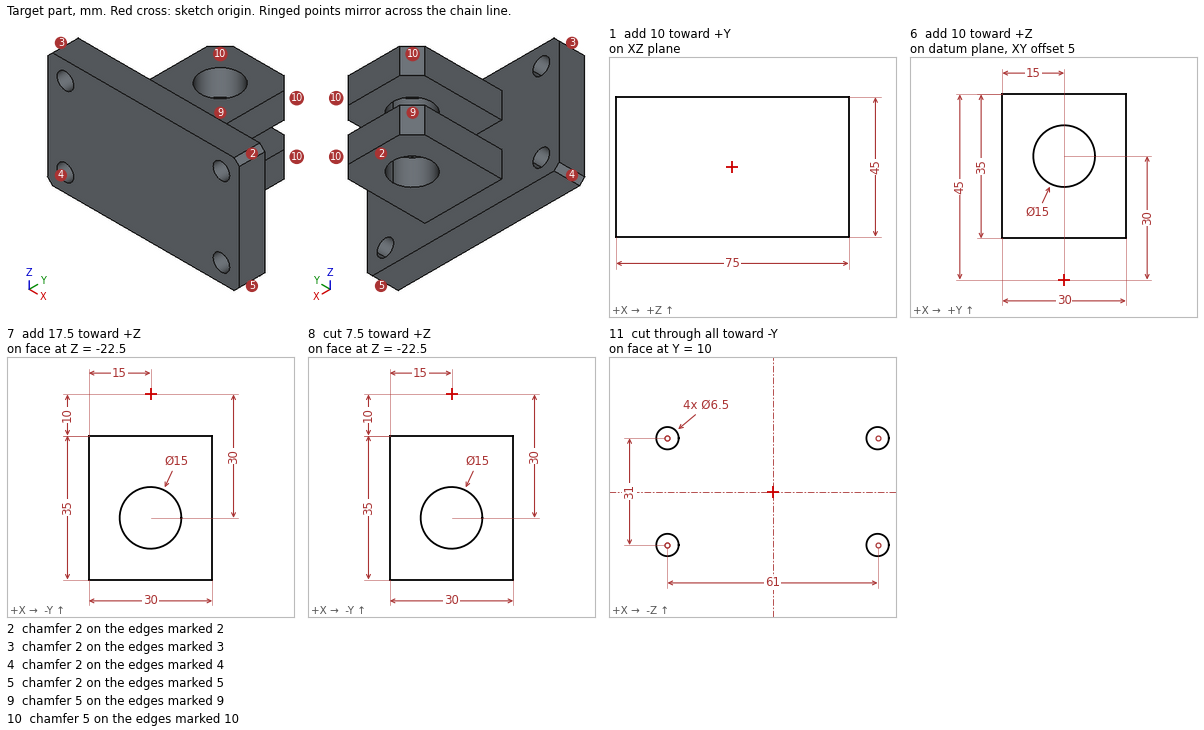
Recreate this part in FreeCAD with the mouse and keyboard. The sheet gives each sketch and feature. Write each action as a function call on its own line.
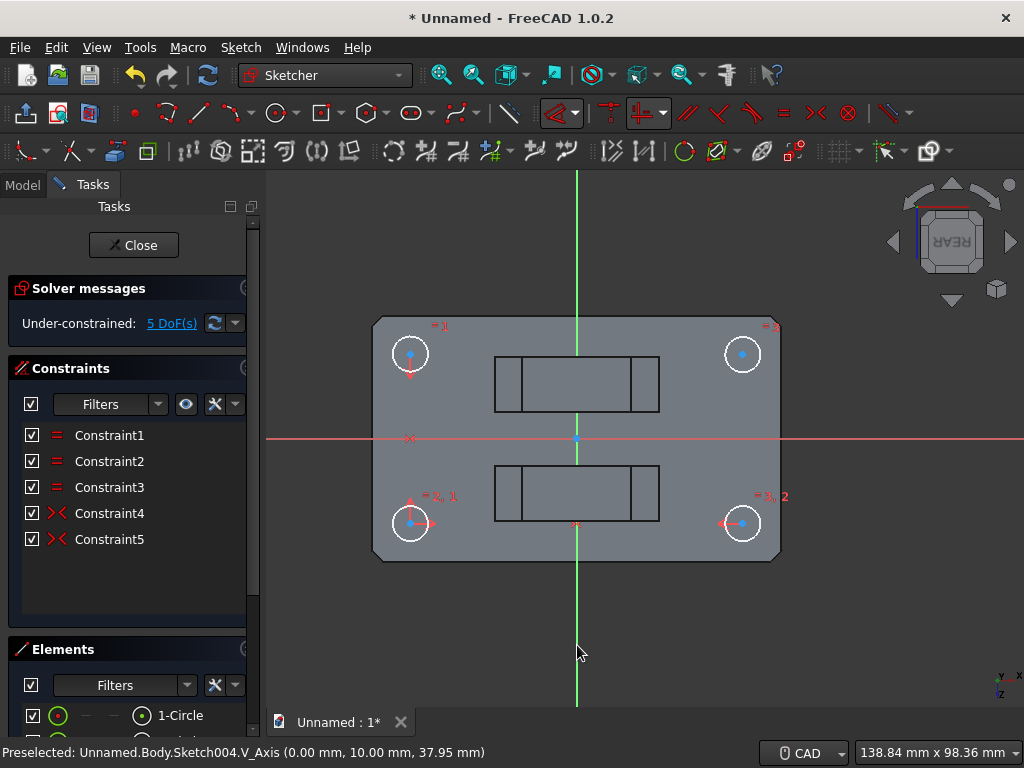
click(410, 354)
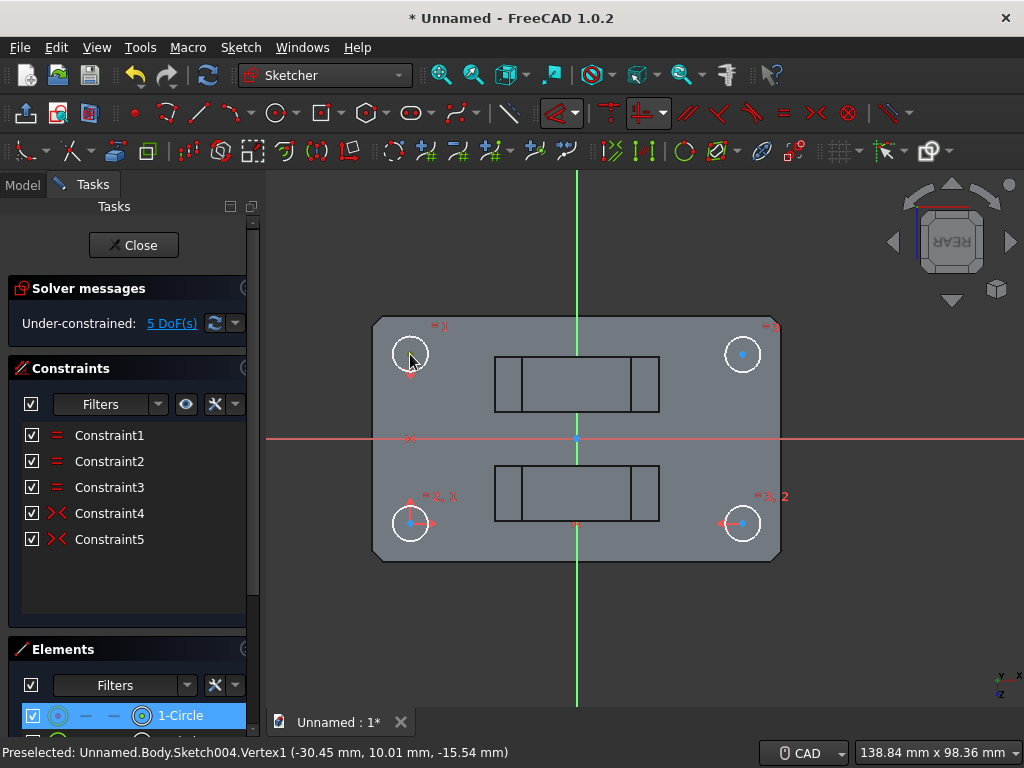
click(743, 355)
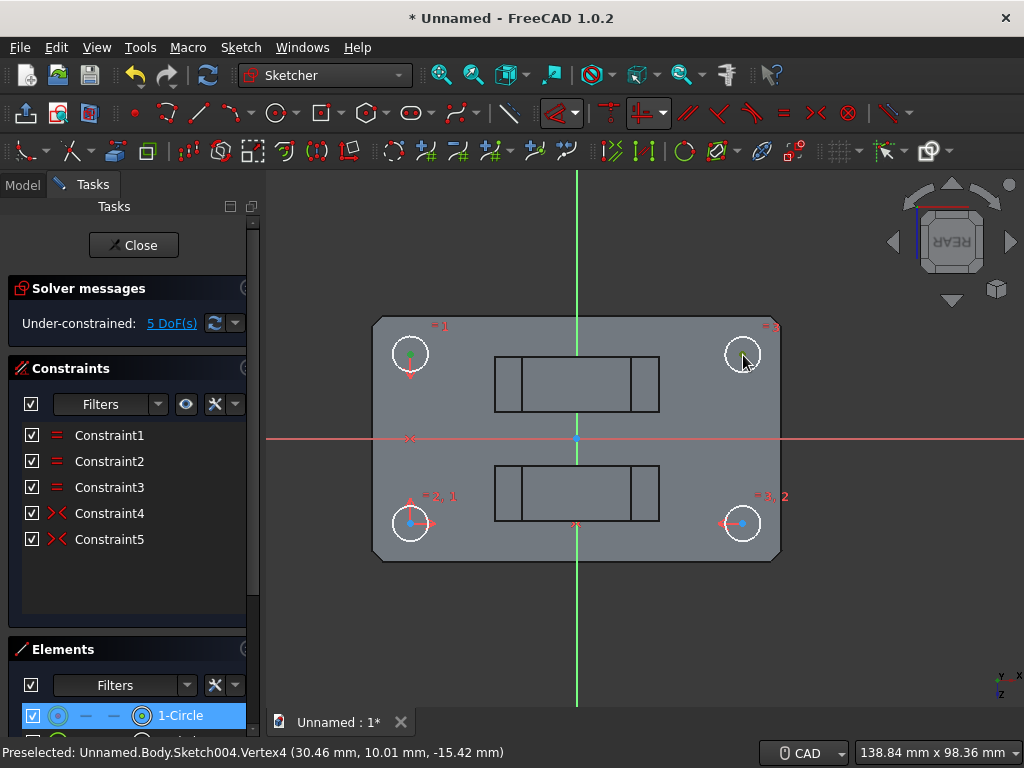
click(577, 645)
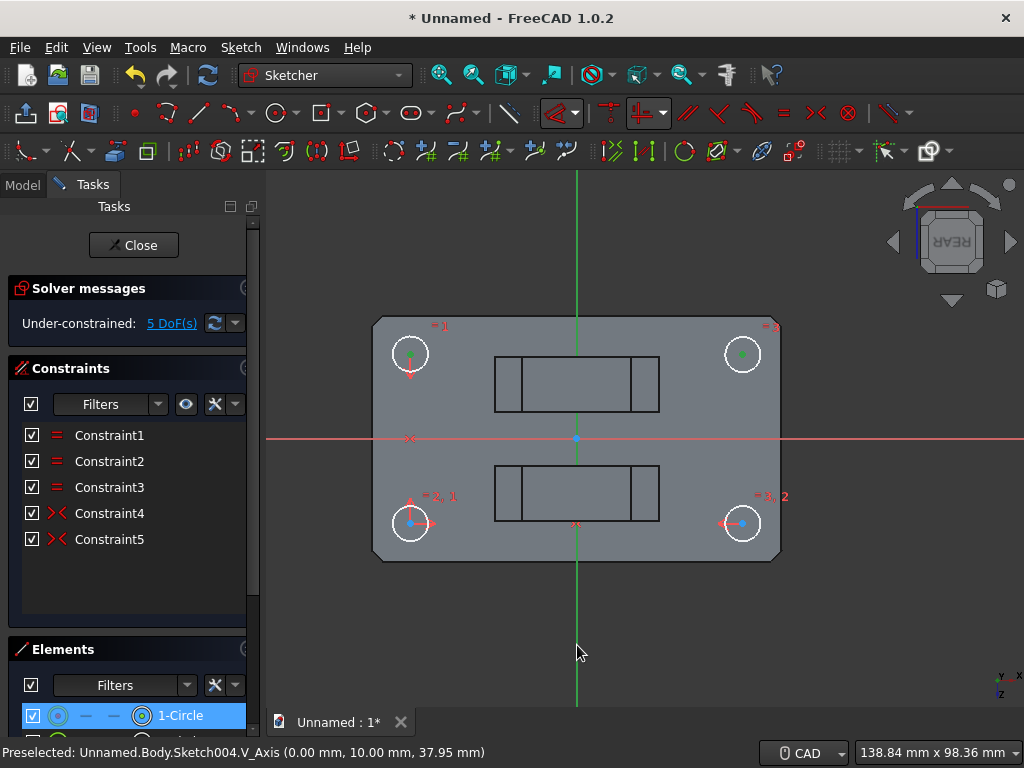
key(s)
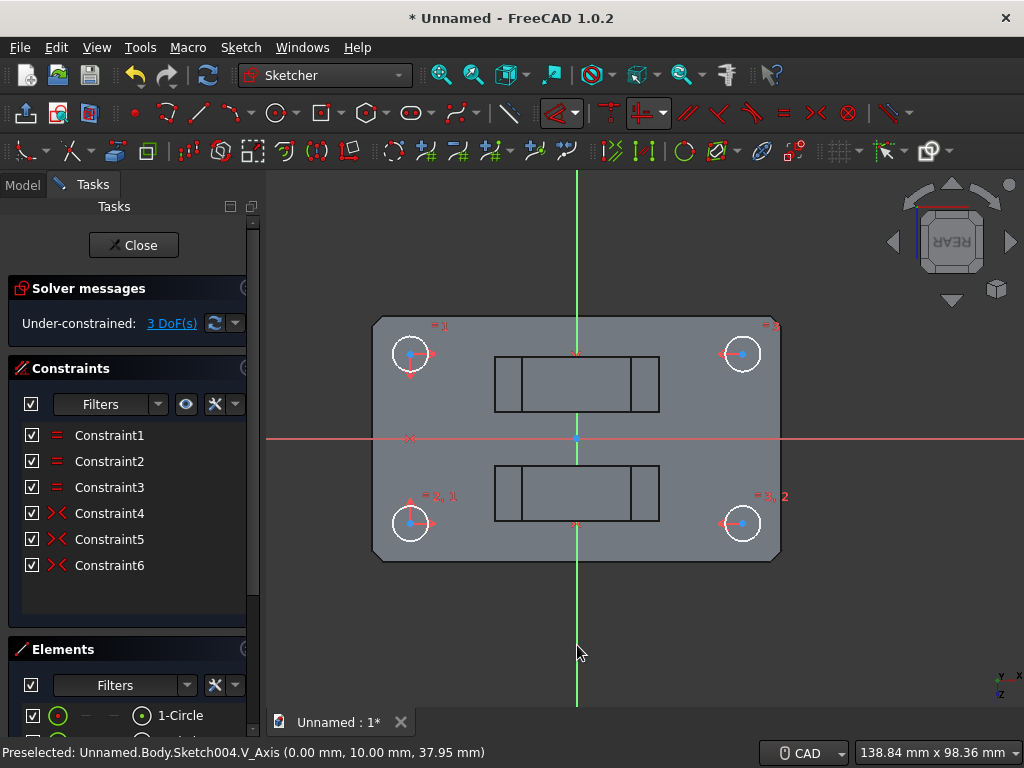
key(d)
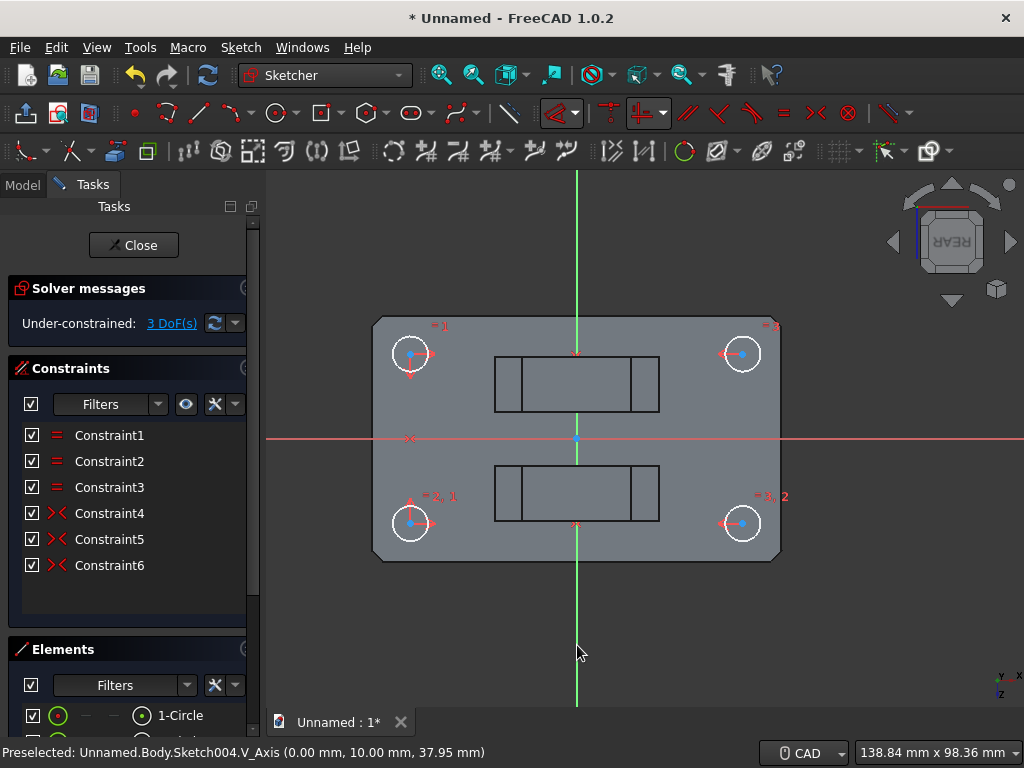
click(423, 342)
click(446, 320)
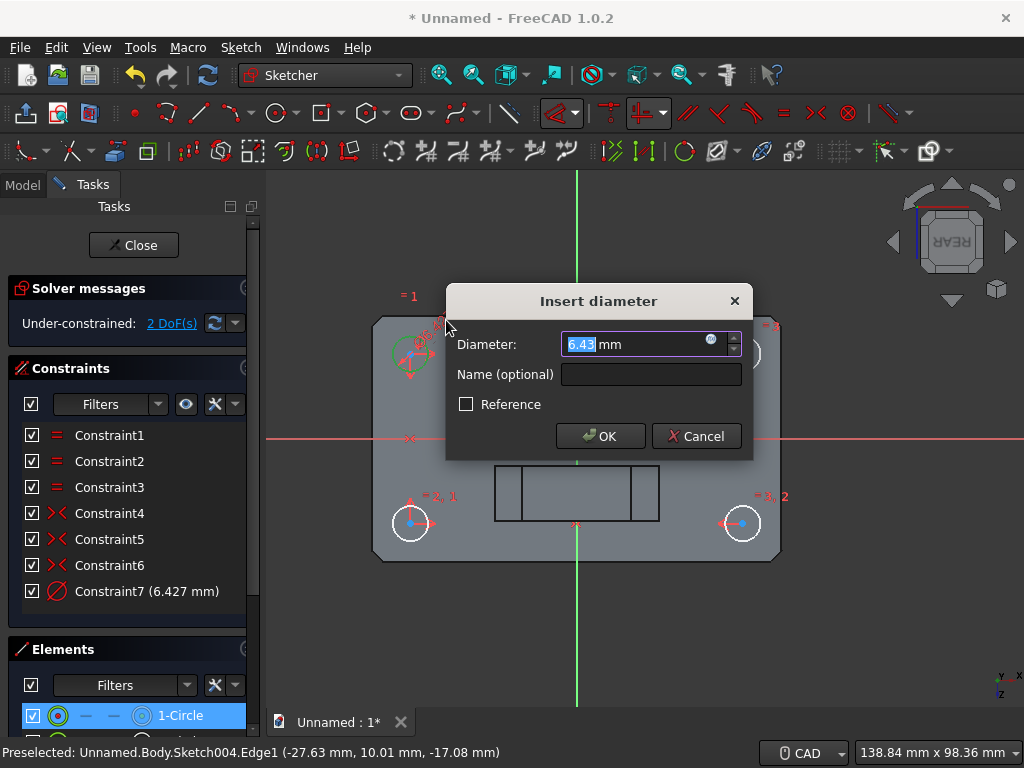
text(6.5)
key(Return)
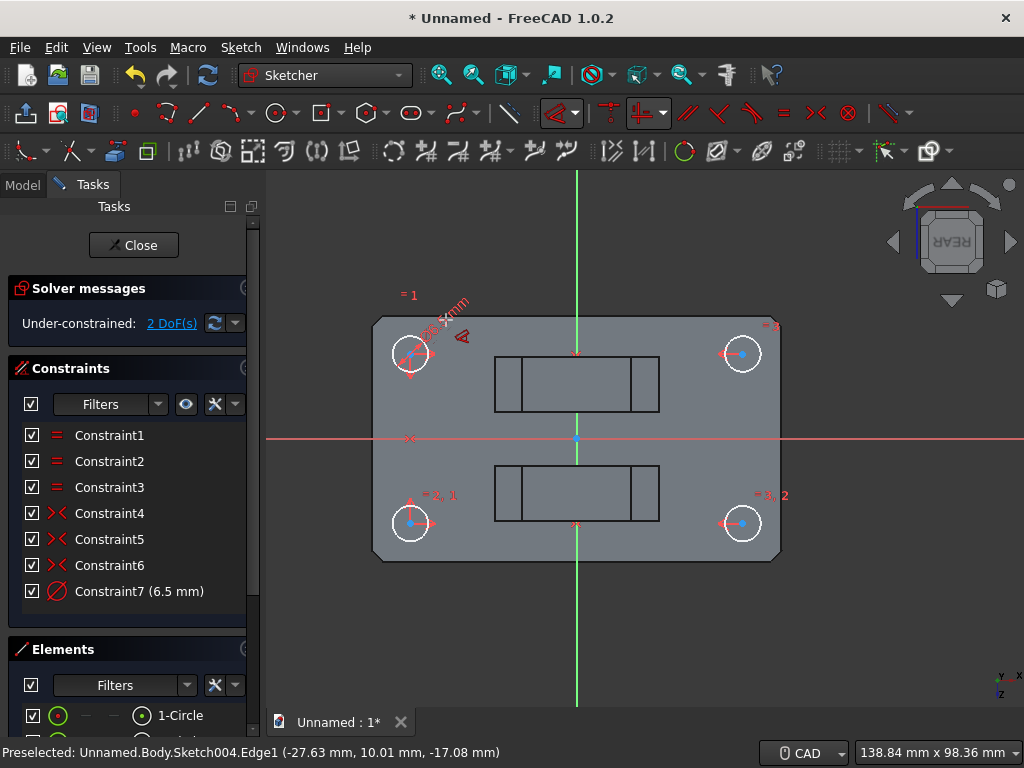
click(410, 354)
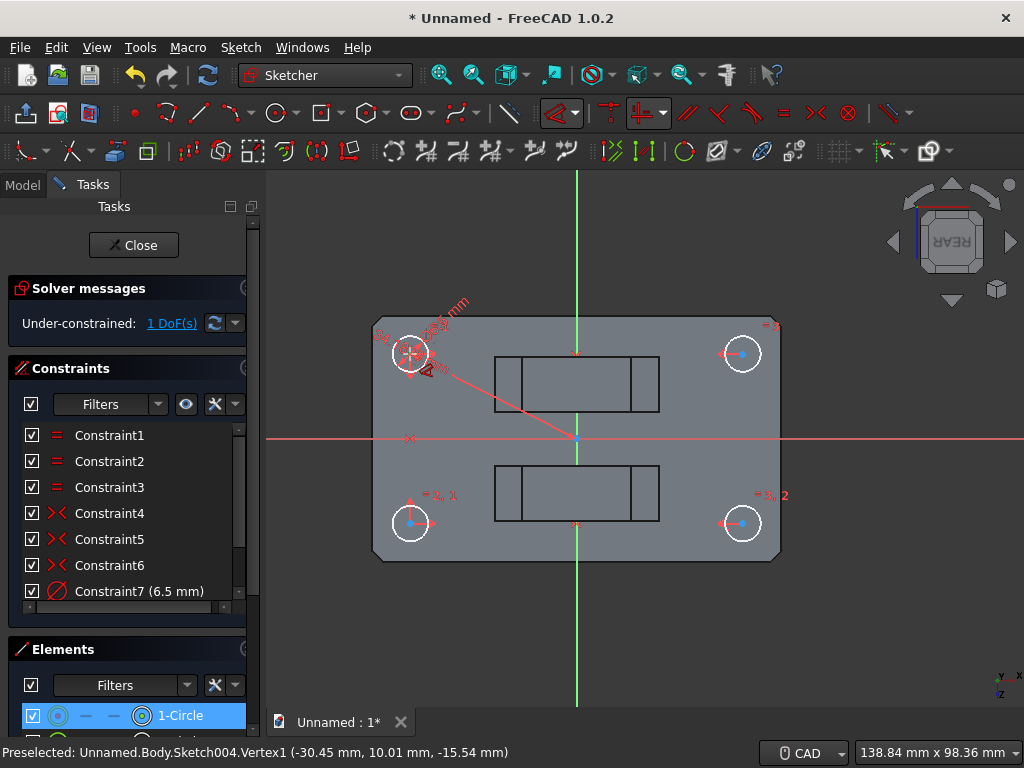
click(410, 524)
click(376, 400)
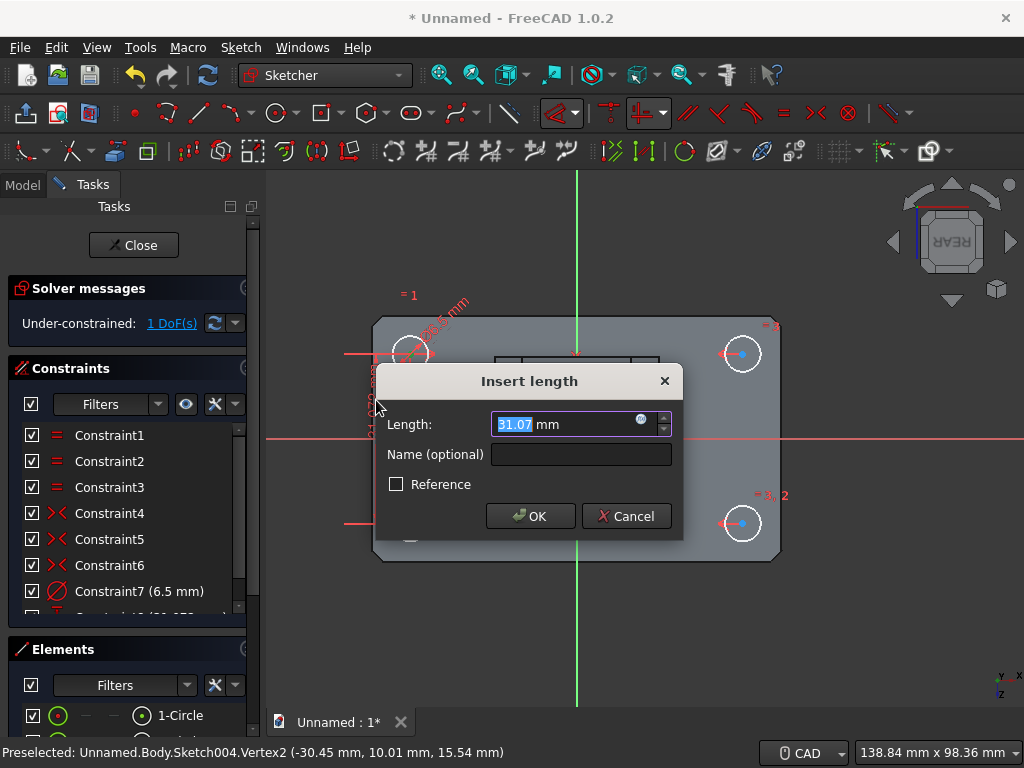
text(31)
key(Return)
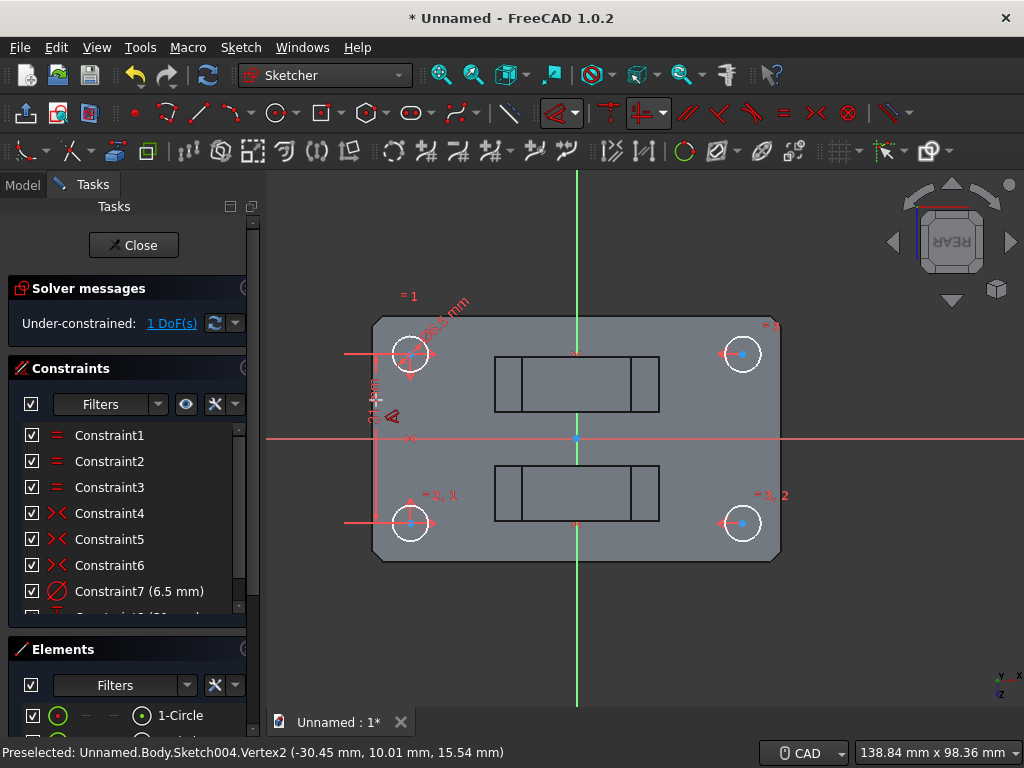
click(410, 523)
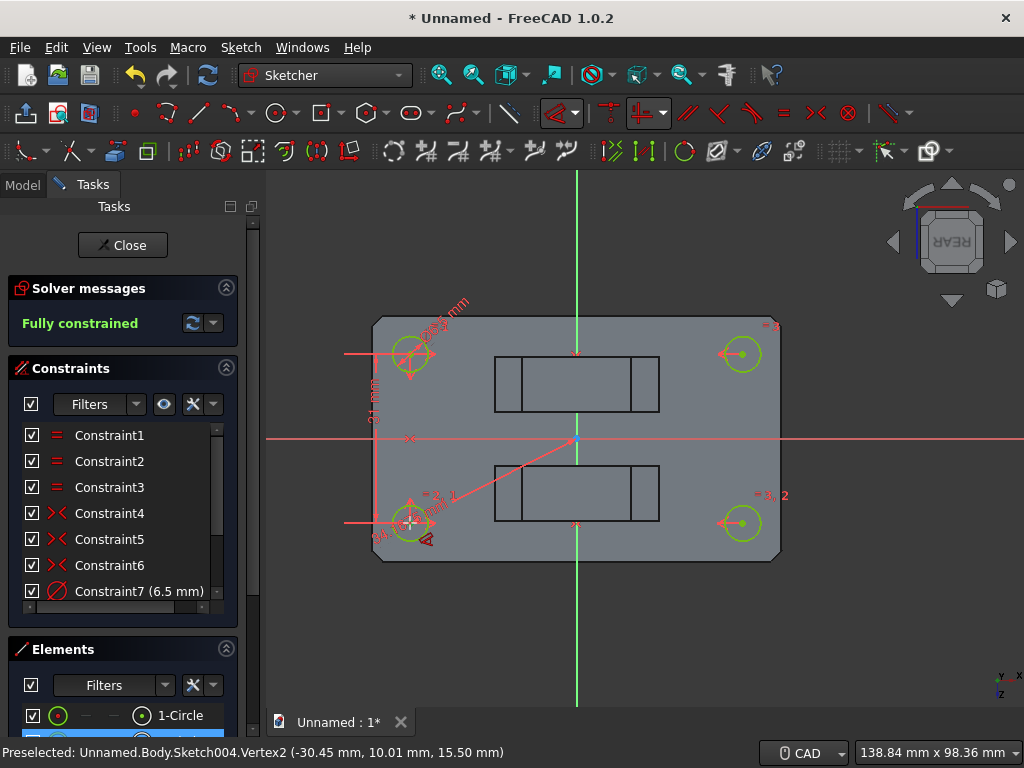
click(743, 523)
click(500, 557)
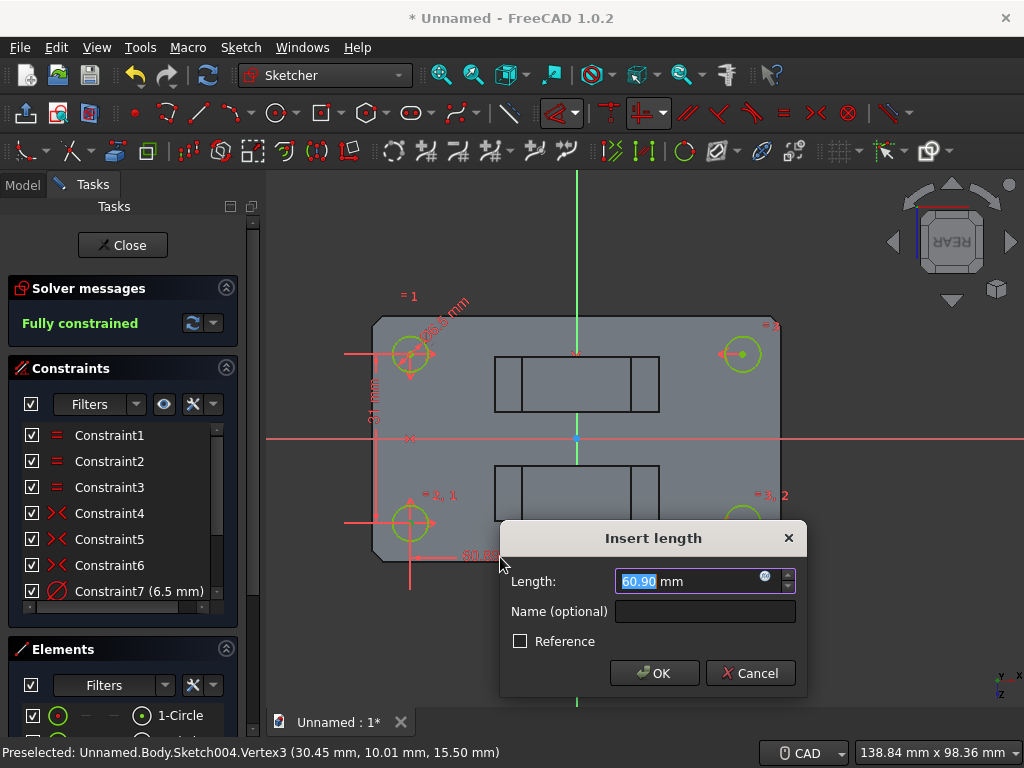
text(61)
key(Return)
key(Escape)